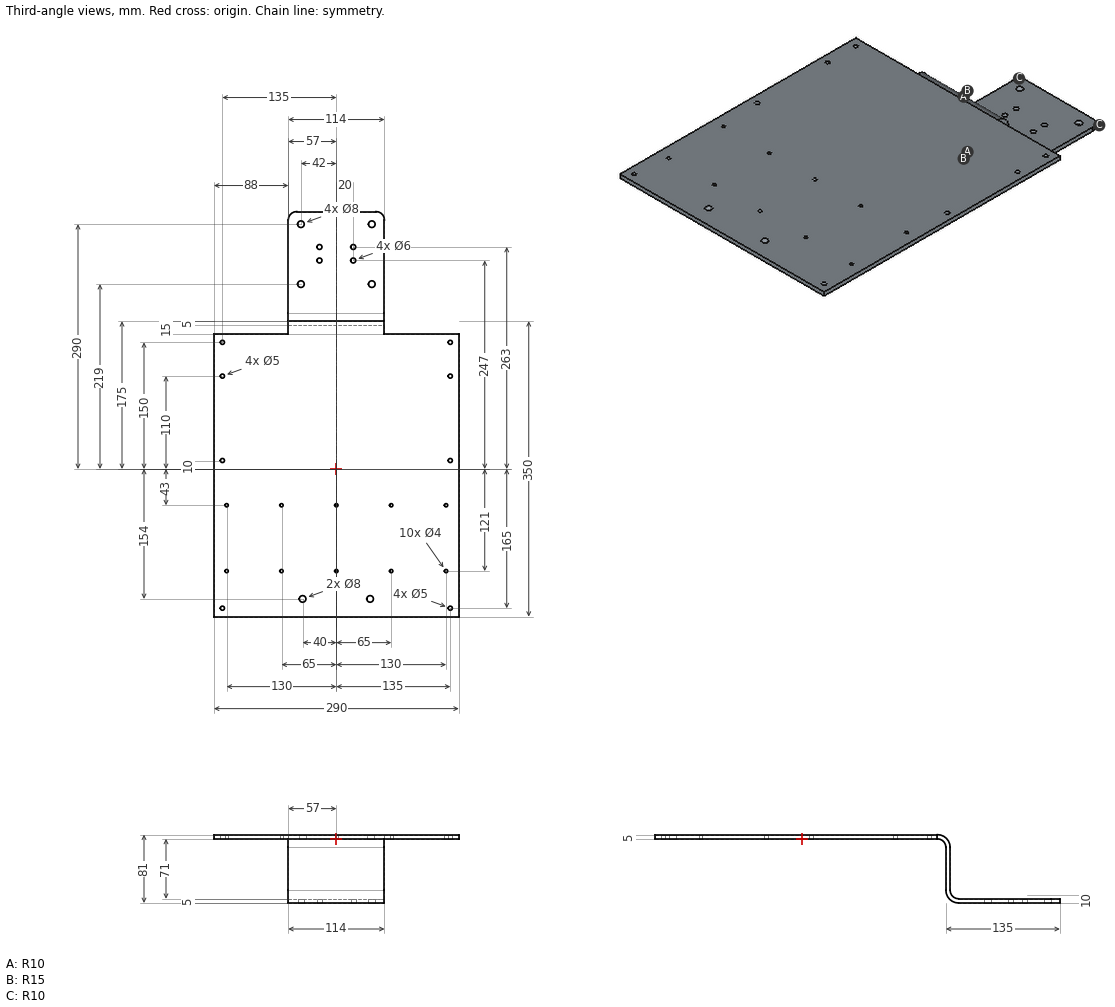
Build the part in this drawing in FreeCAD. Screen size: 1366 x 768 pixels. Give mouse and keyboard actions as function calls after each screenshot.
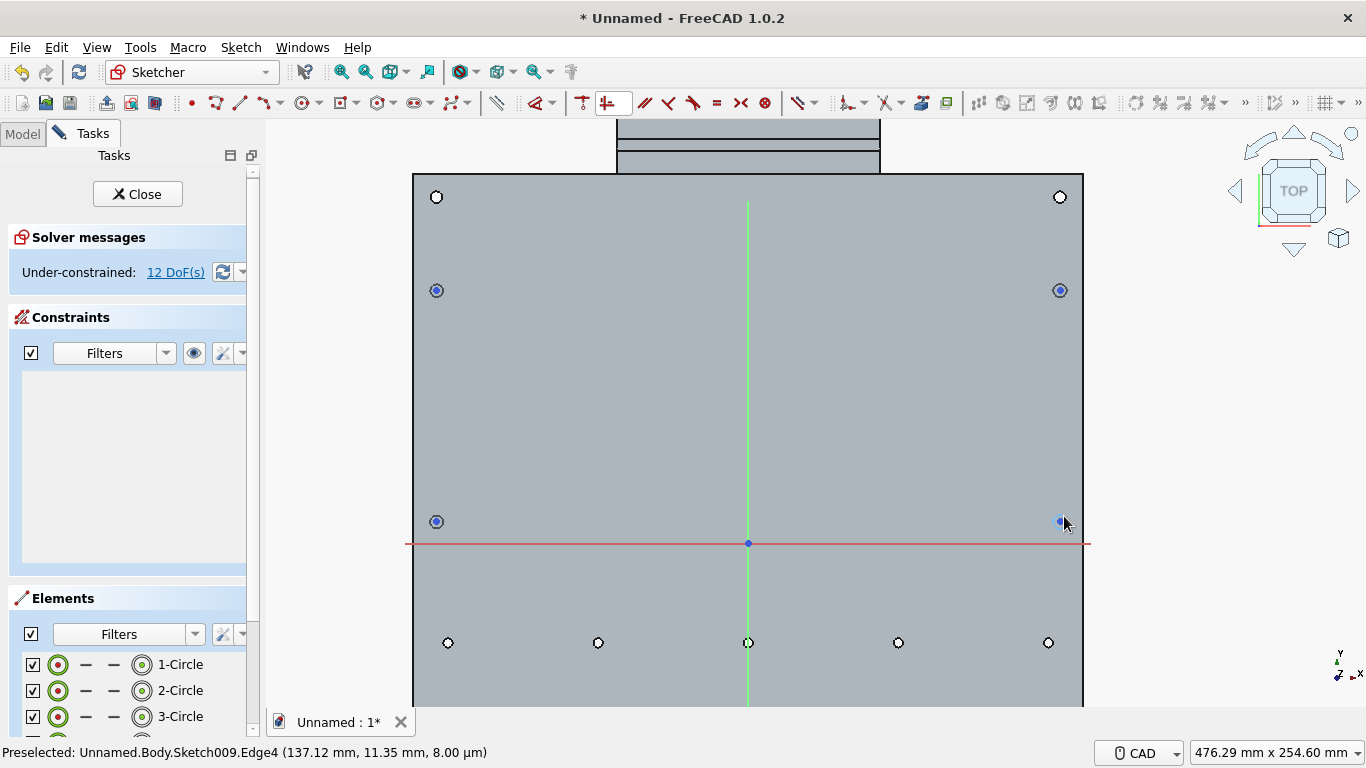
scroll(441, 286, up, 4)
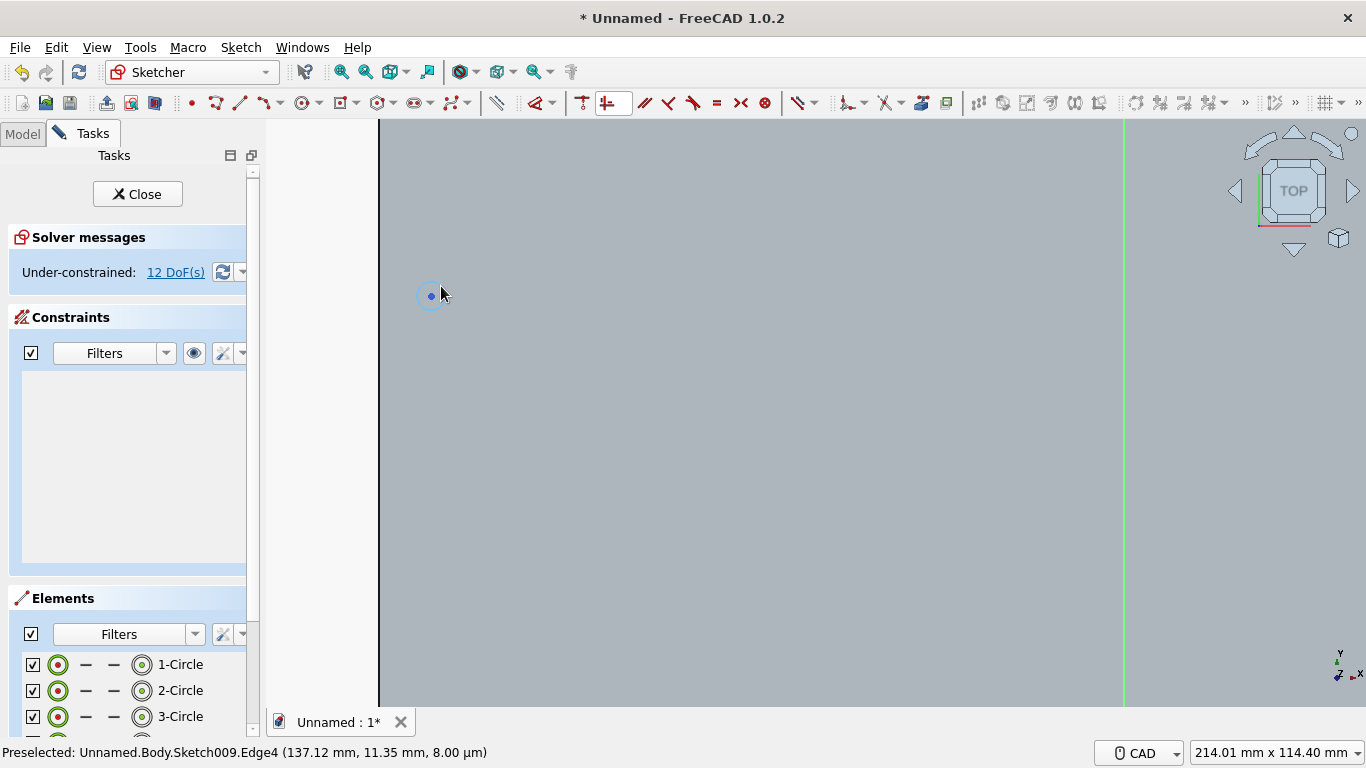
click(441, 286)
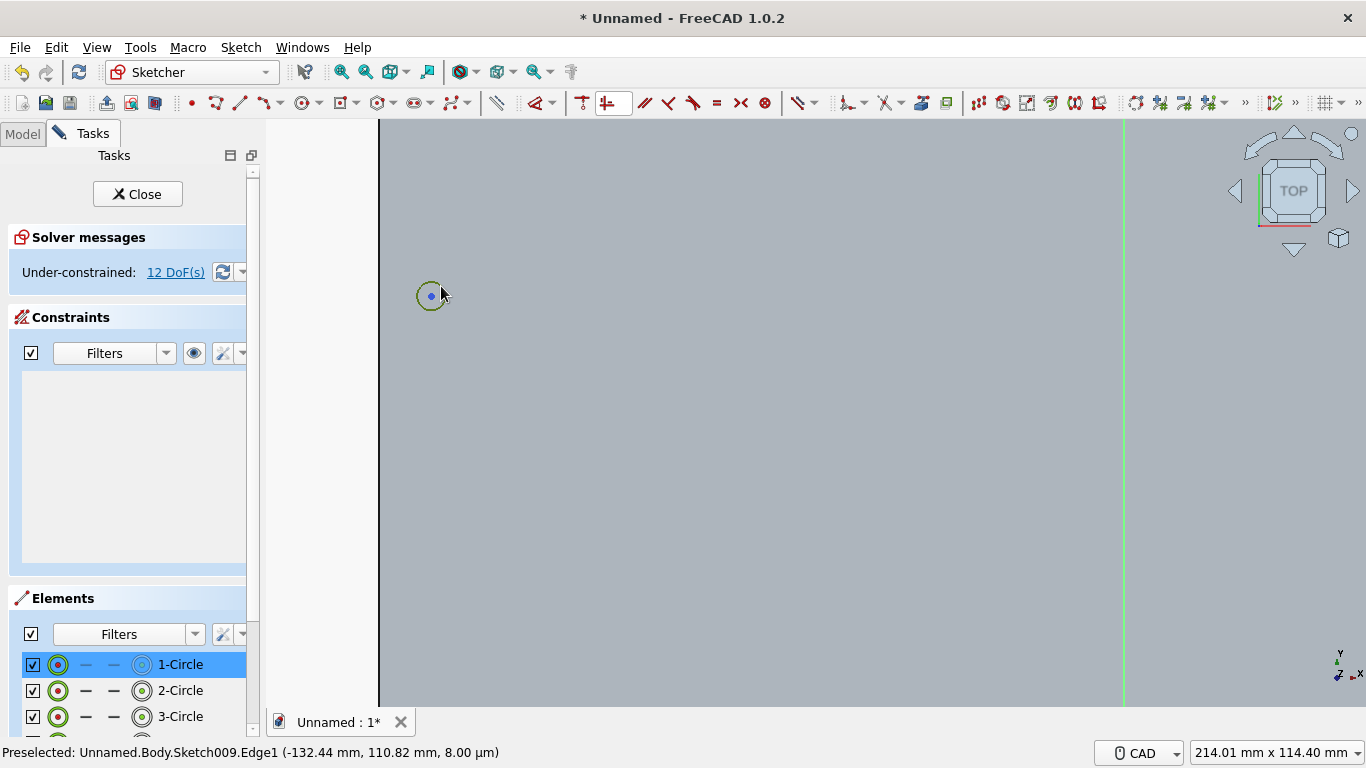
scroll(440, 285, down, 4)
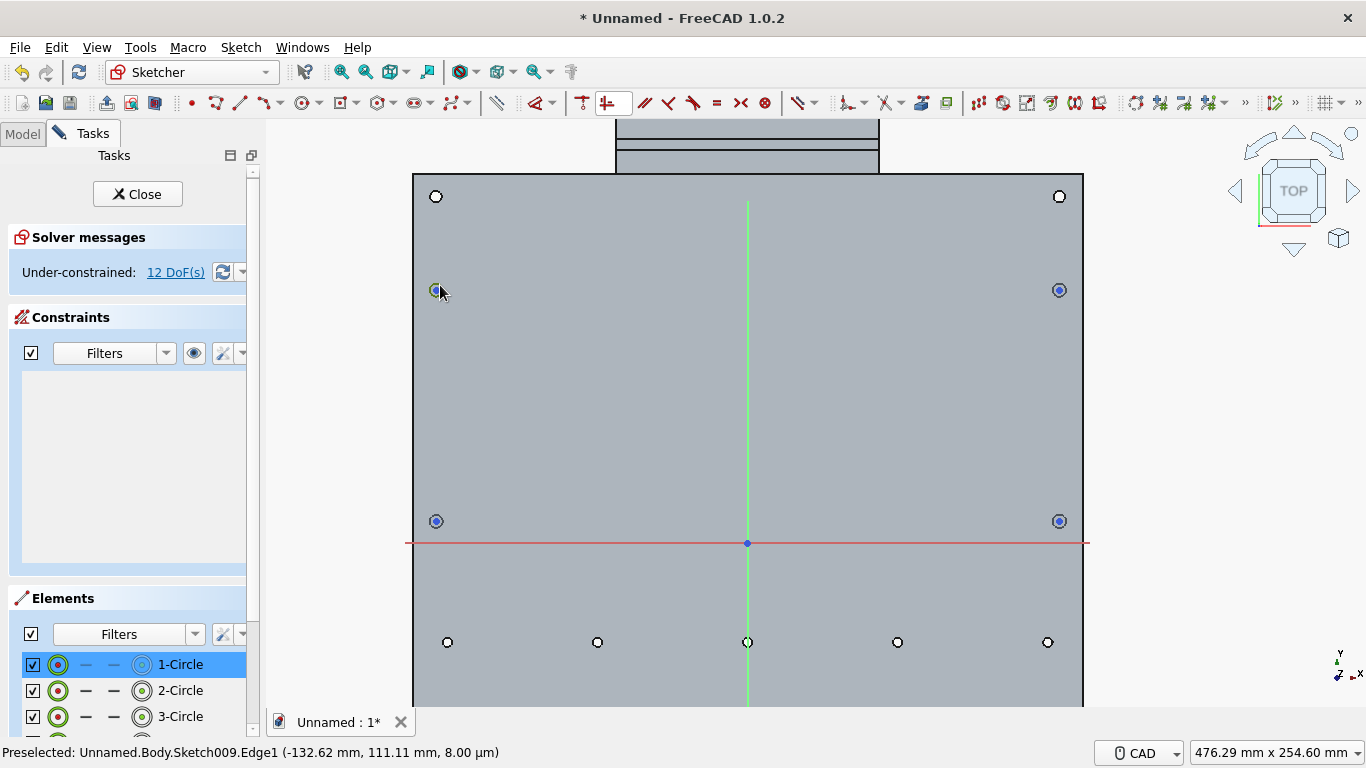
scroll(441, 517, up, 4)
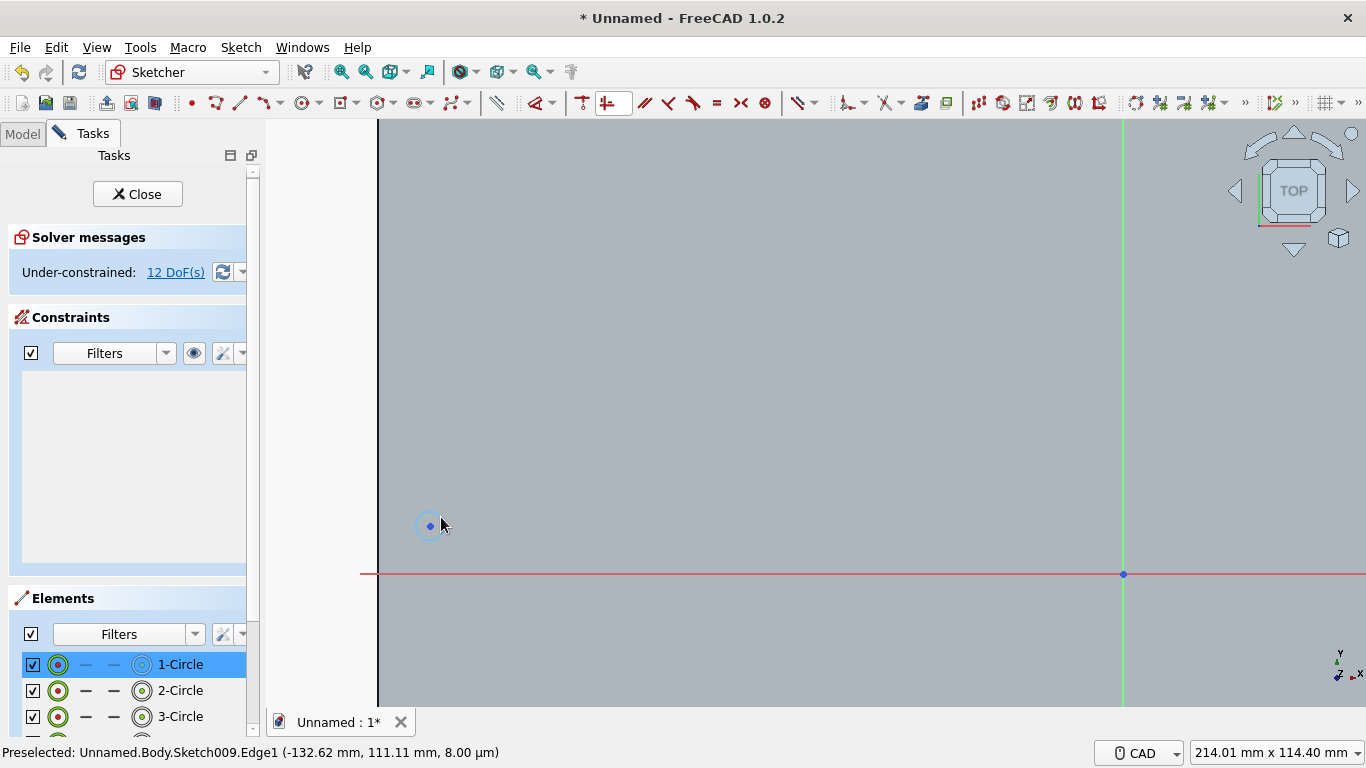
click(440, 516)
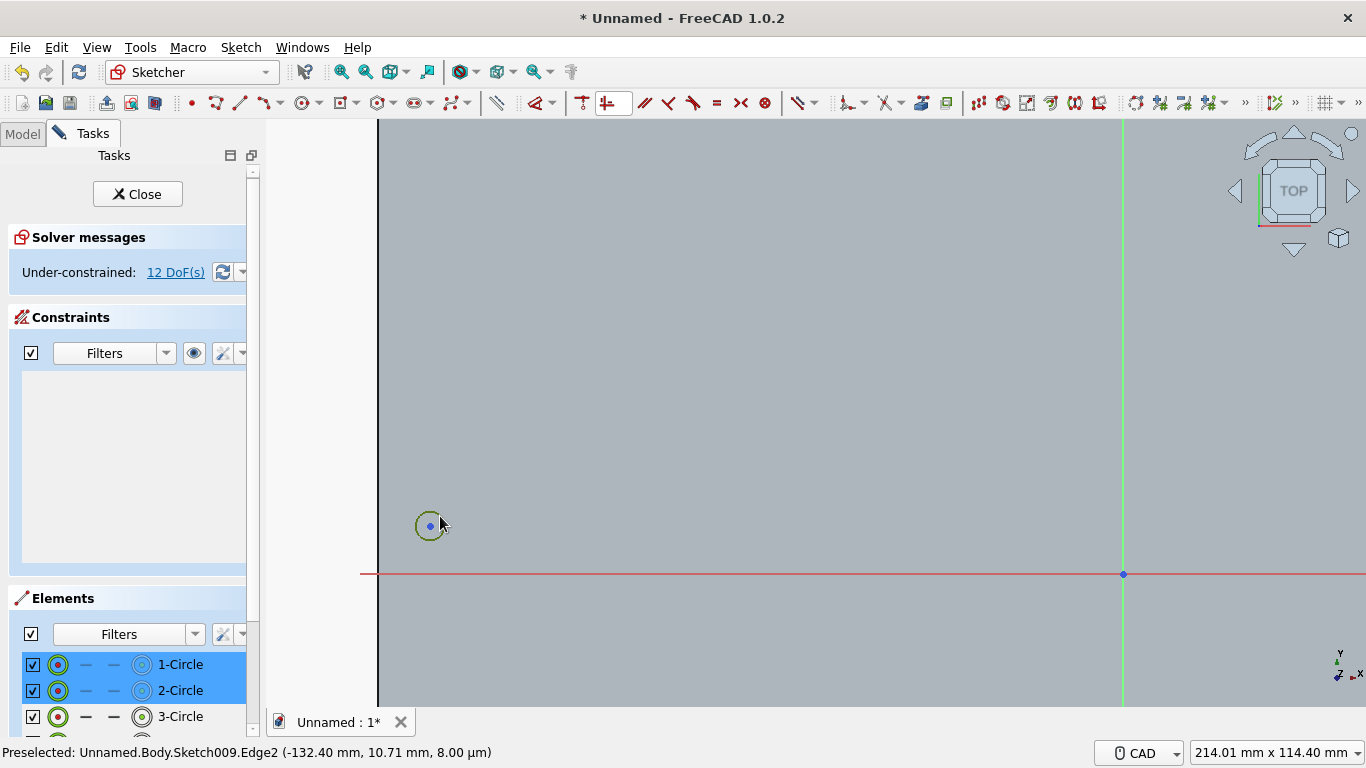
scroll(441, 517, down, 4)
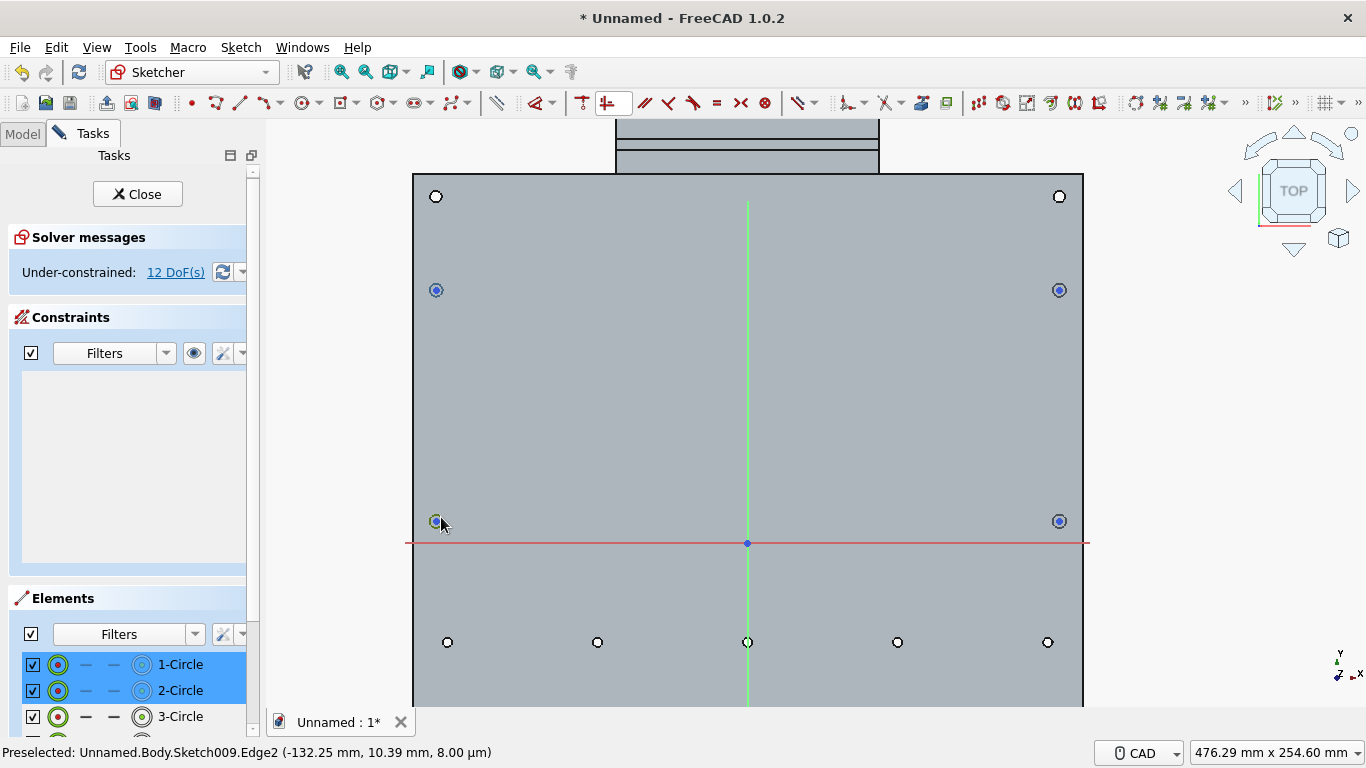
scroll(1064, 286, up, 4)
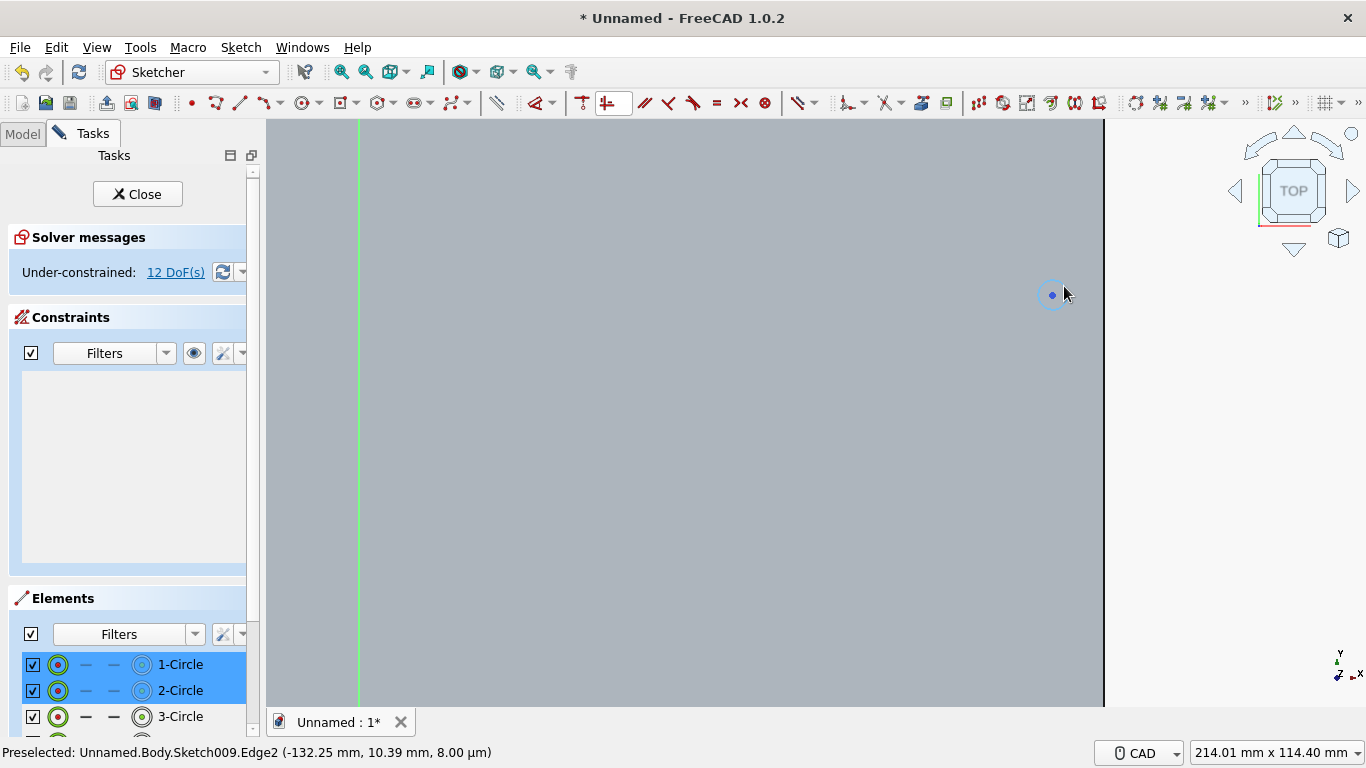
click(1063, 285)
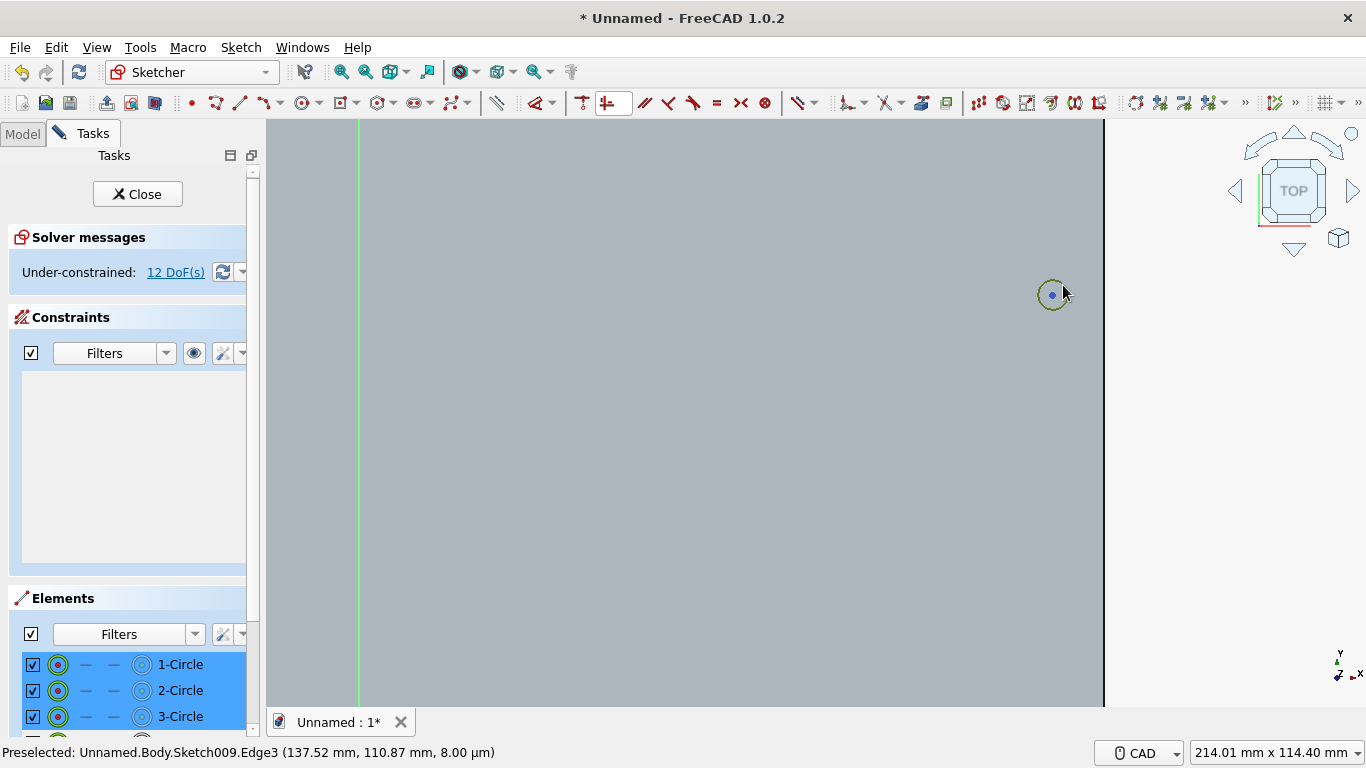
scroll(1064, 286, down, 4)